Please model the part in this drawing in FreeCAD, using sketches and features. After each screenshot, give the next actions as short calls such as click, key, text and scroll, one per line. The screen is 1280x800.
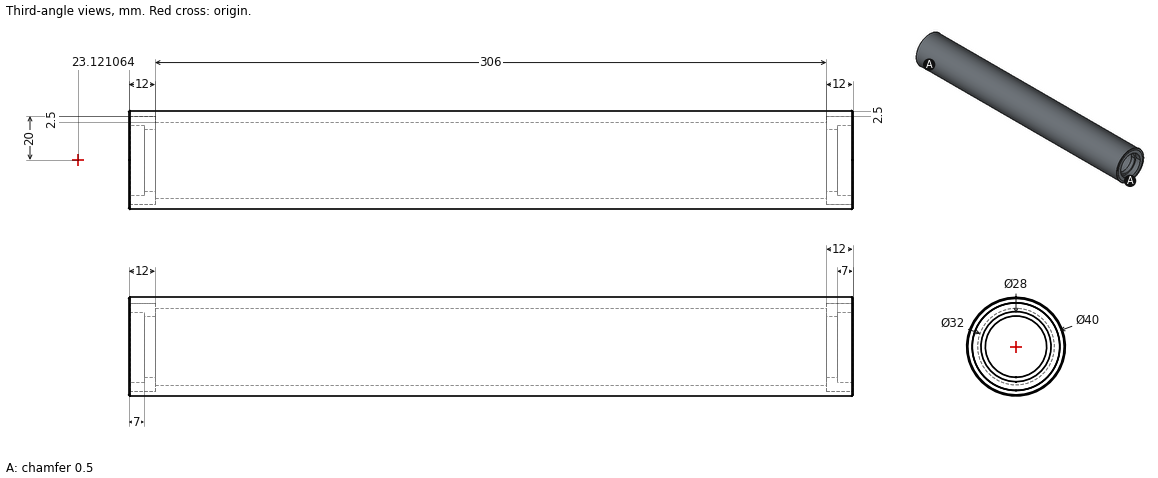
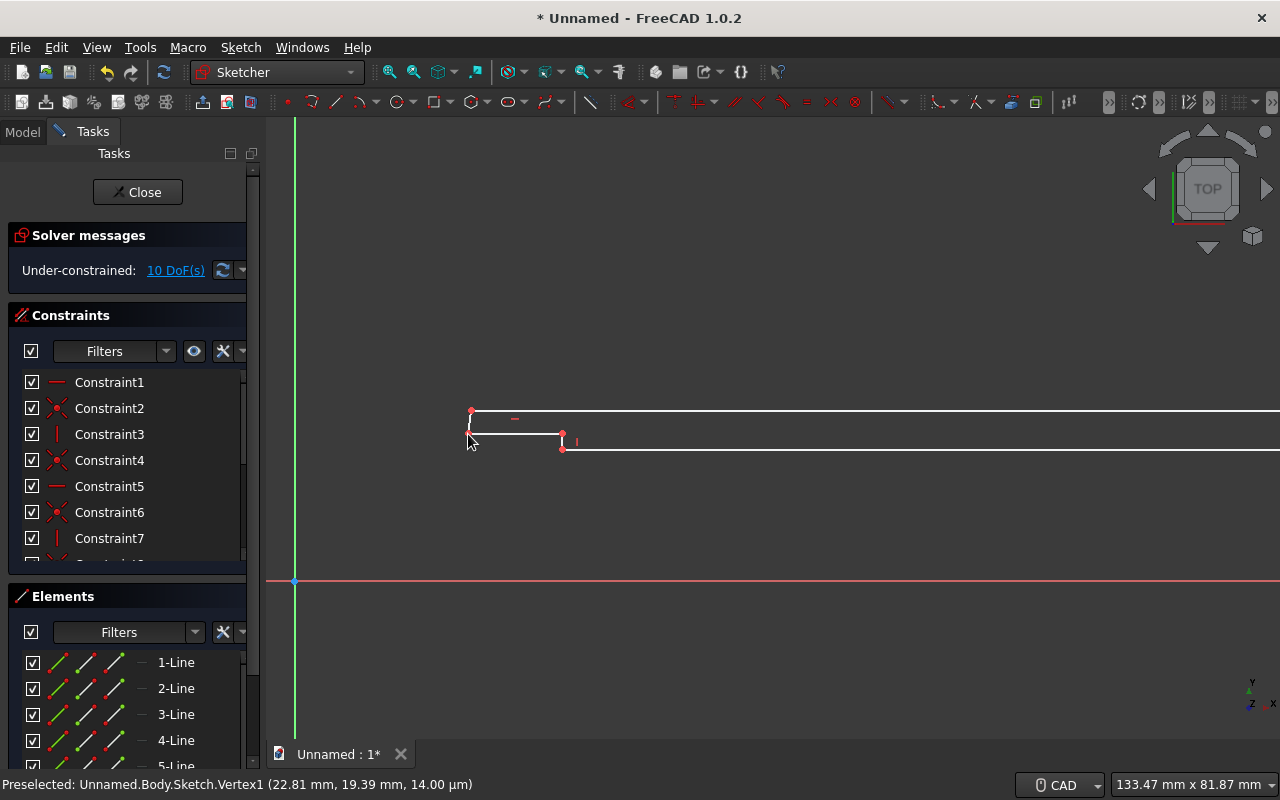
scroll(469, 411, down, 8)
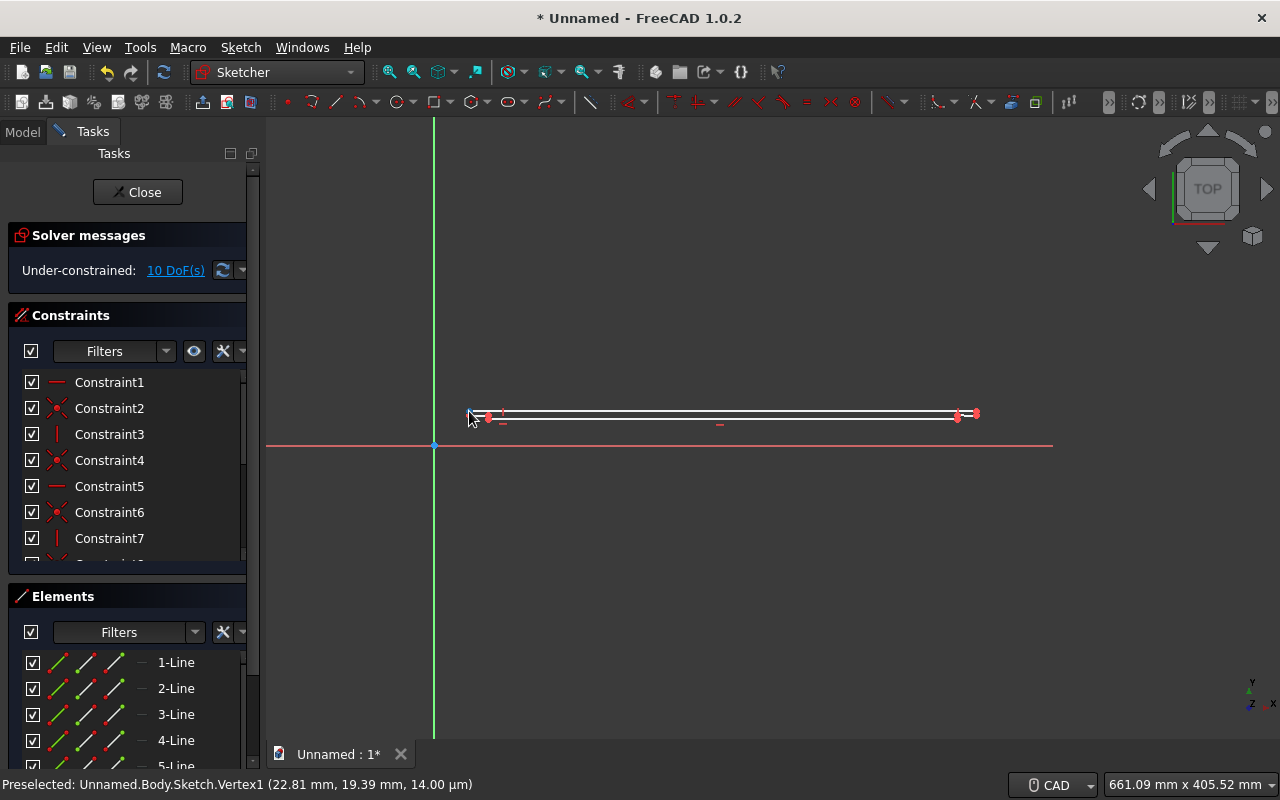
scroll(963, 415, up, 7)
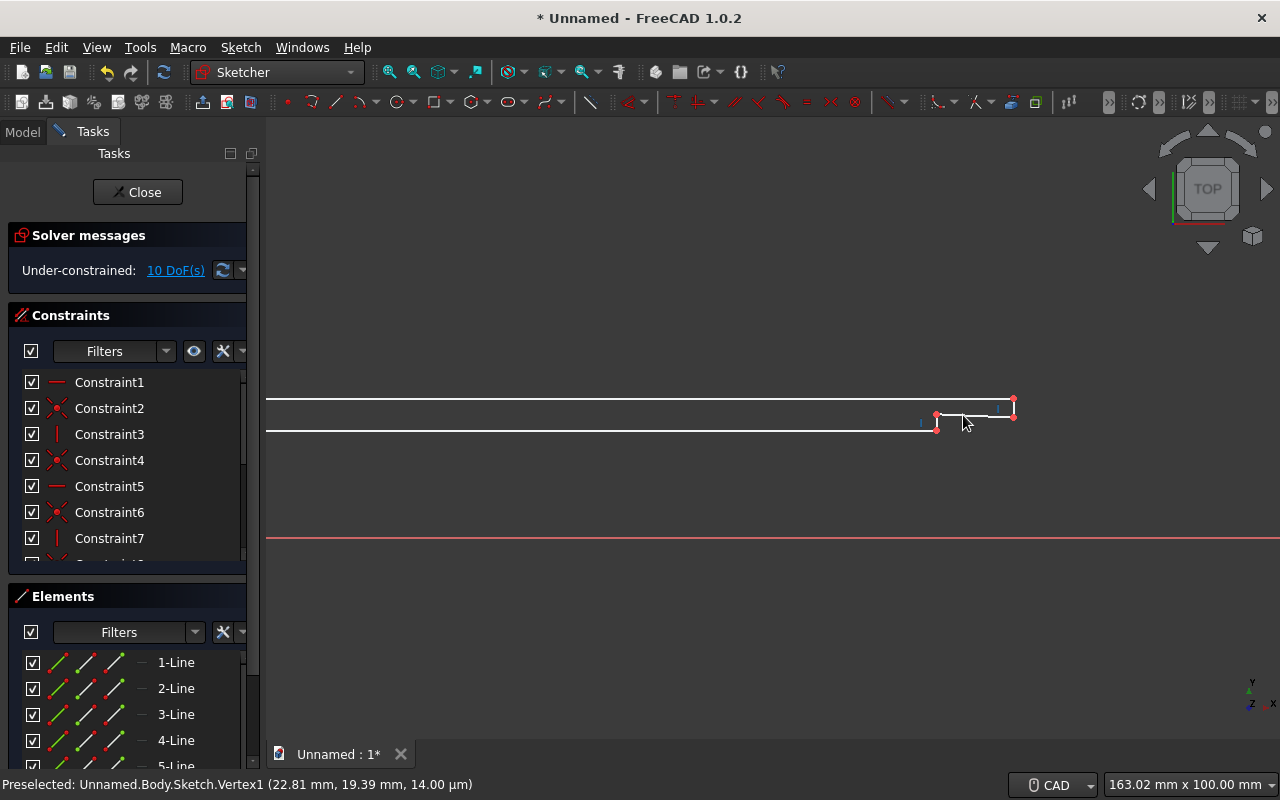
click(960, 415)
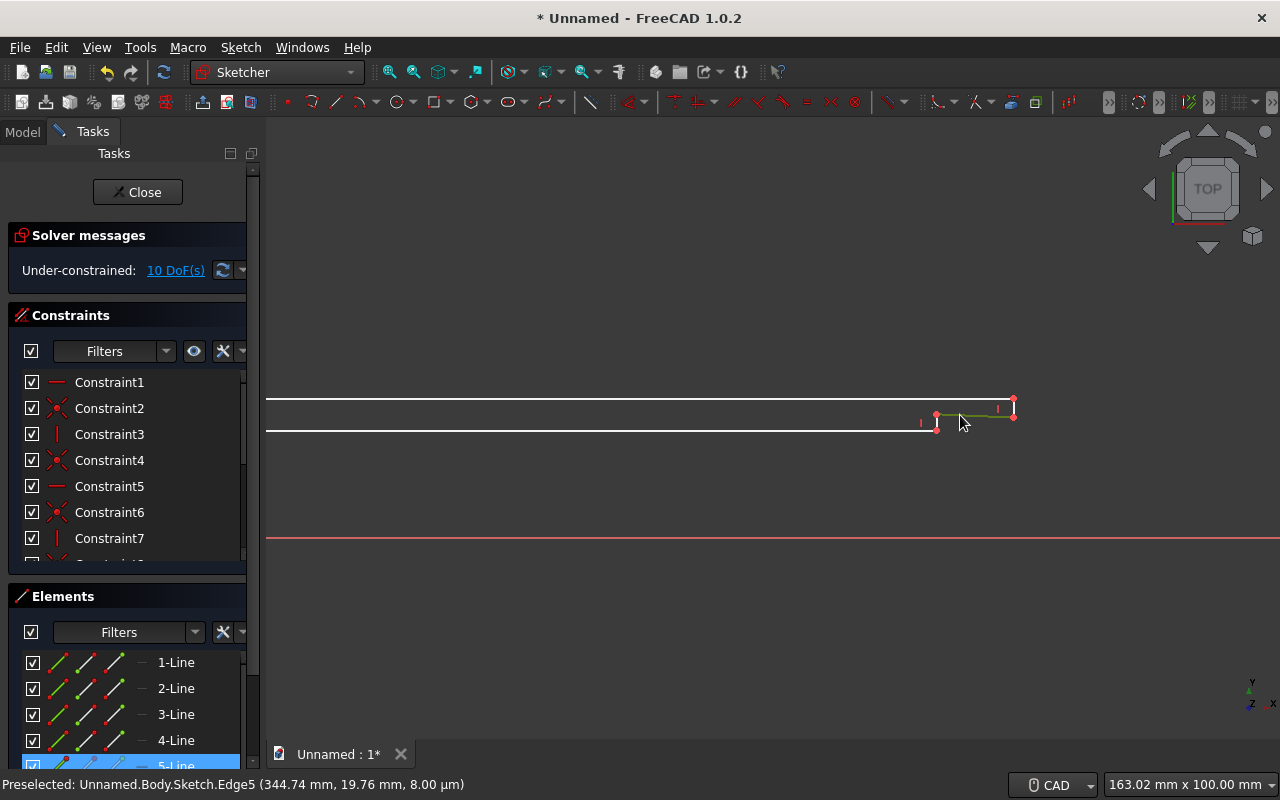
click(716, 102)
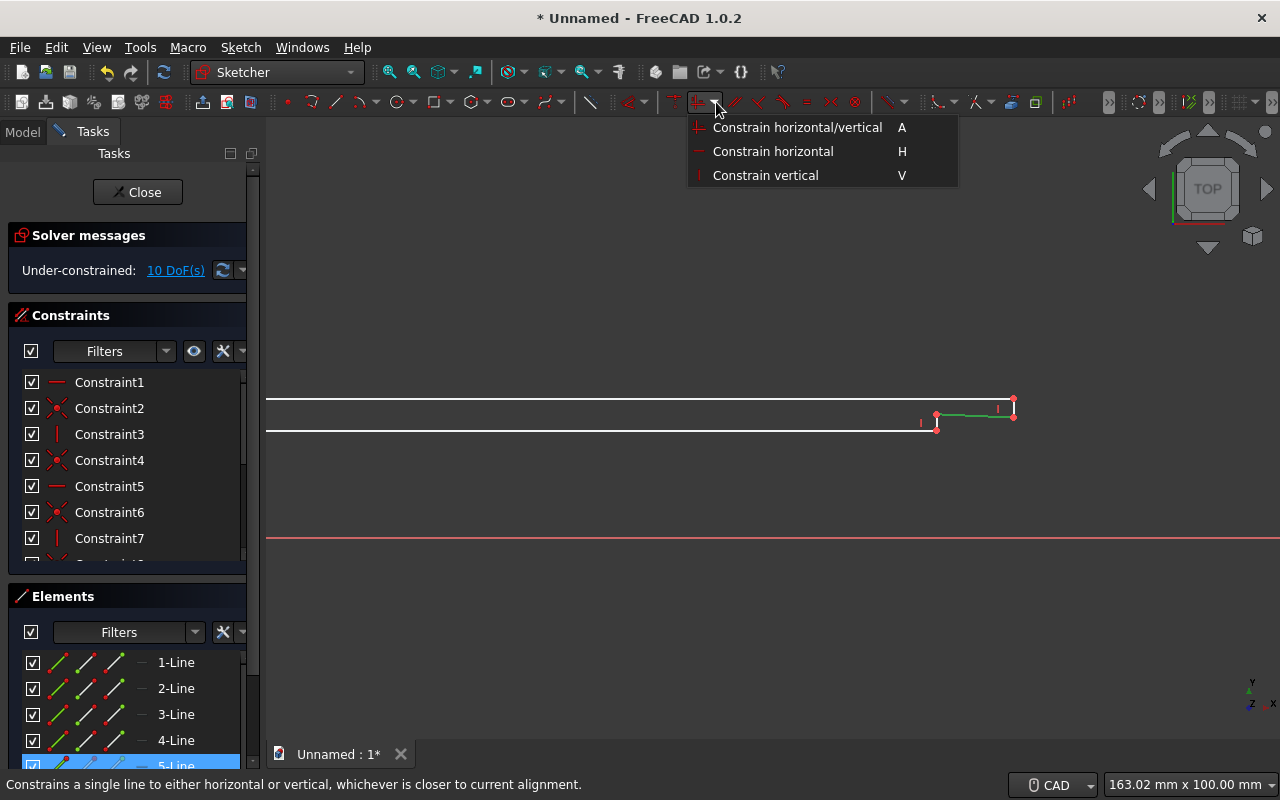
click(823, 151)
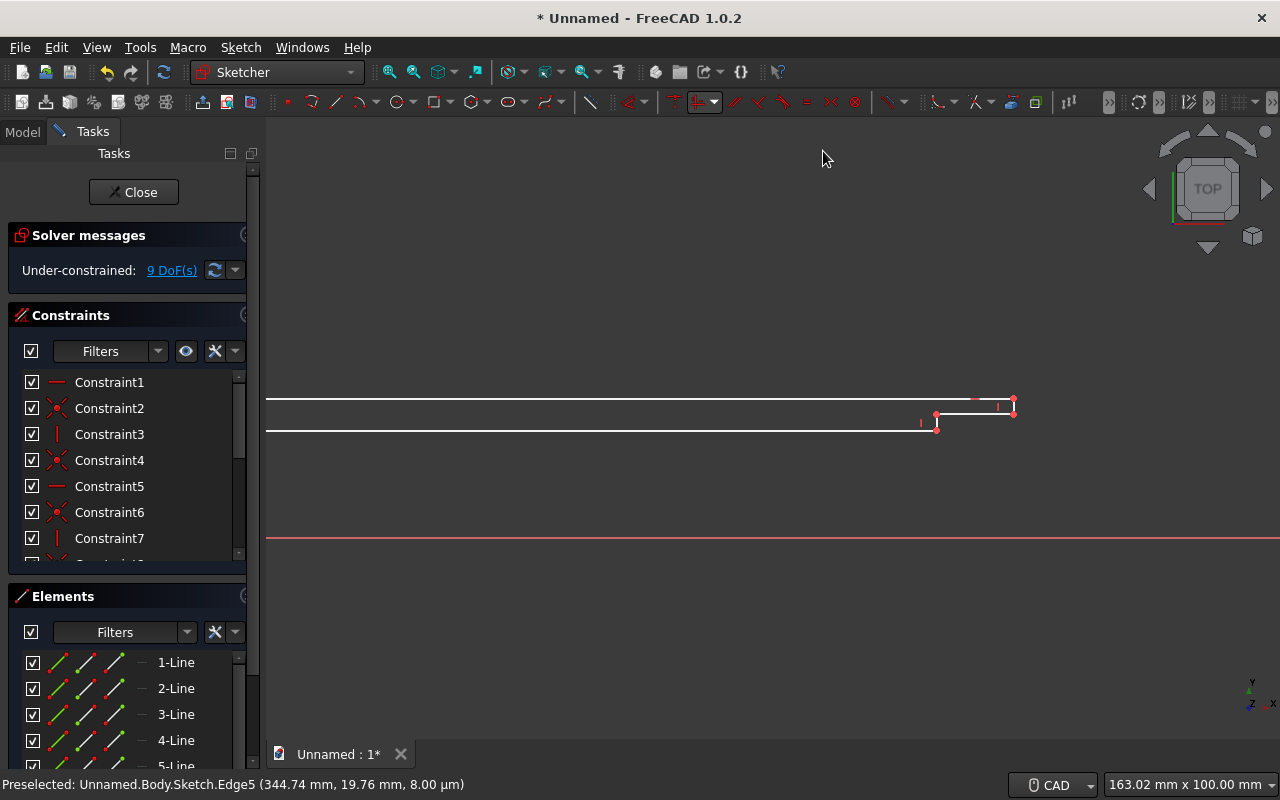
scroll(963, 415, down, 7)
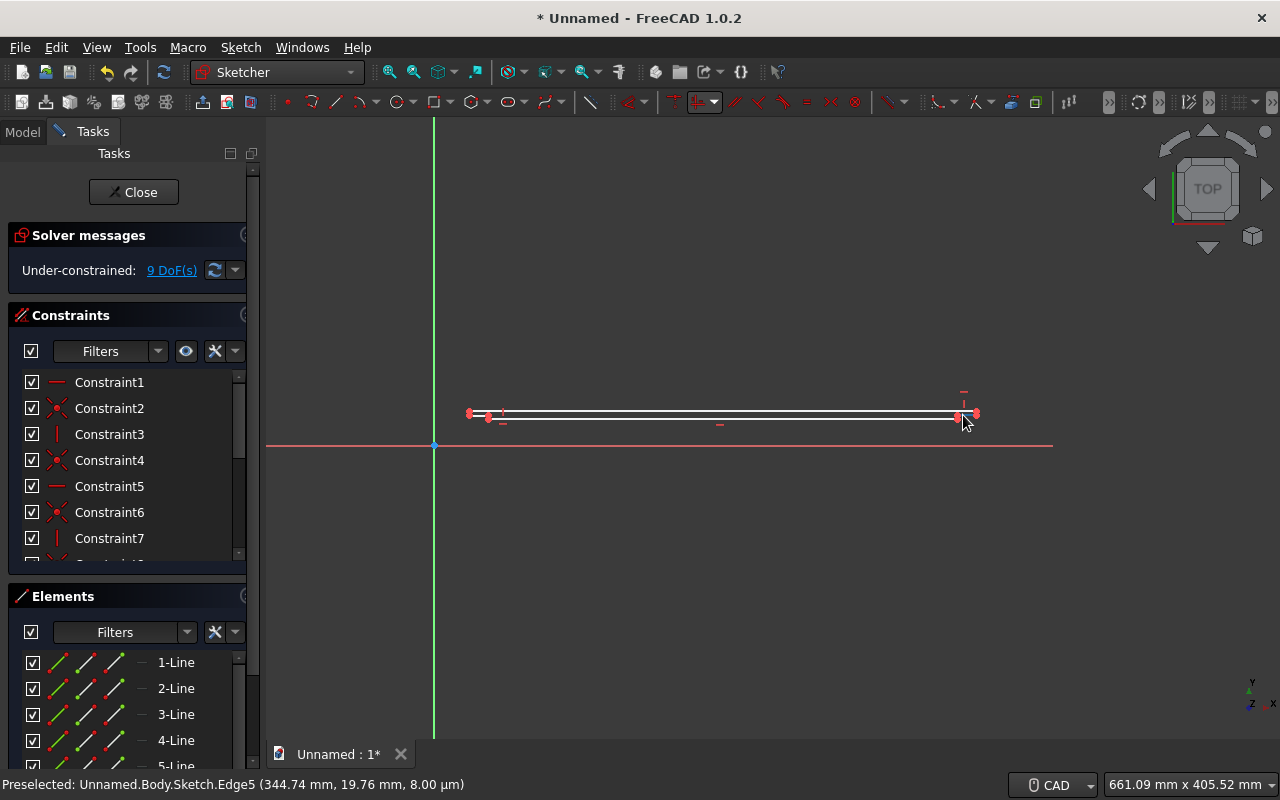
scroll(469, 414, up, 9)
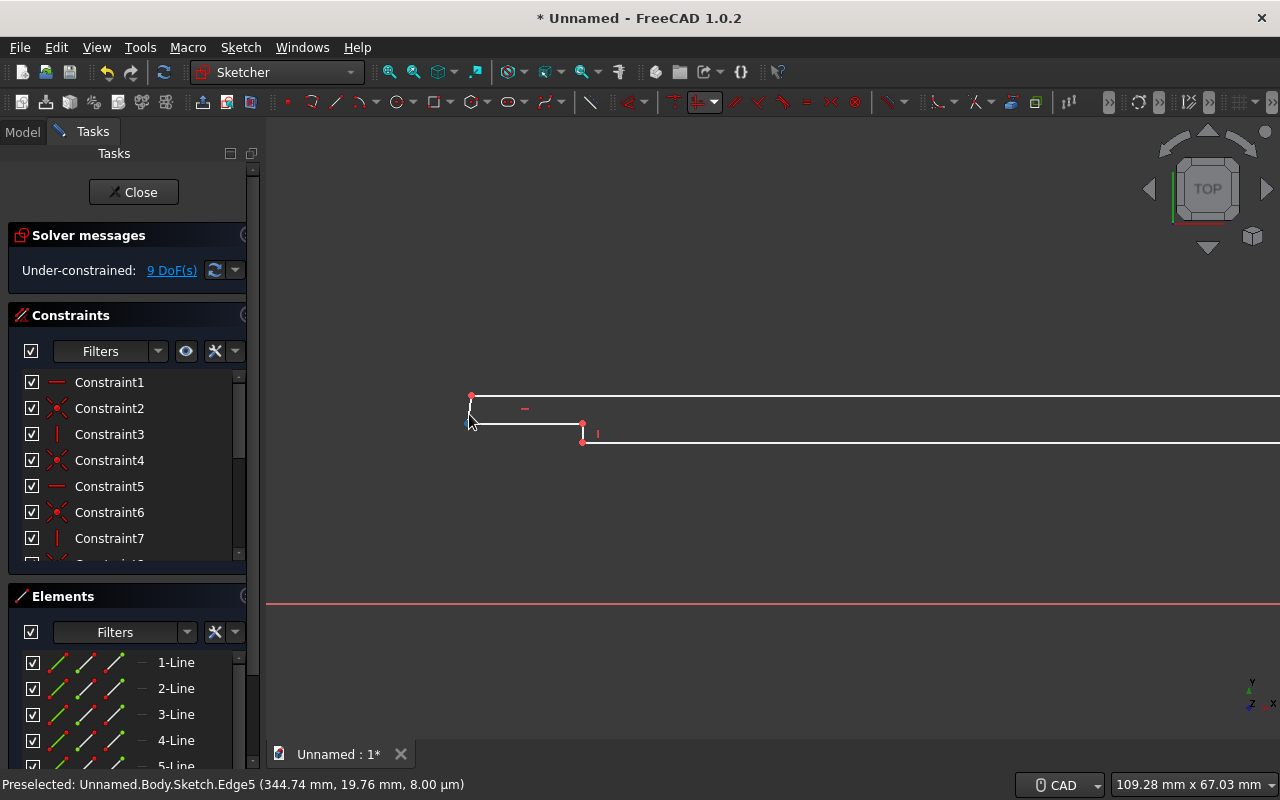
click(470, 410)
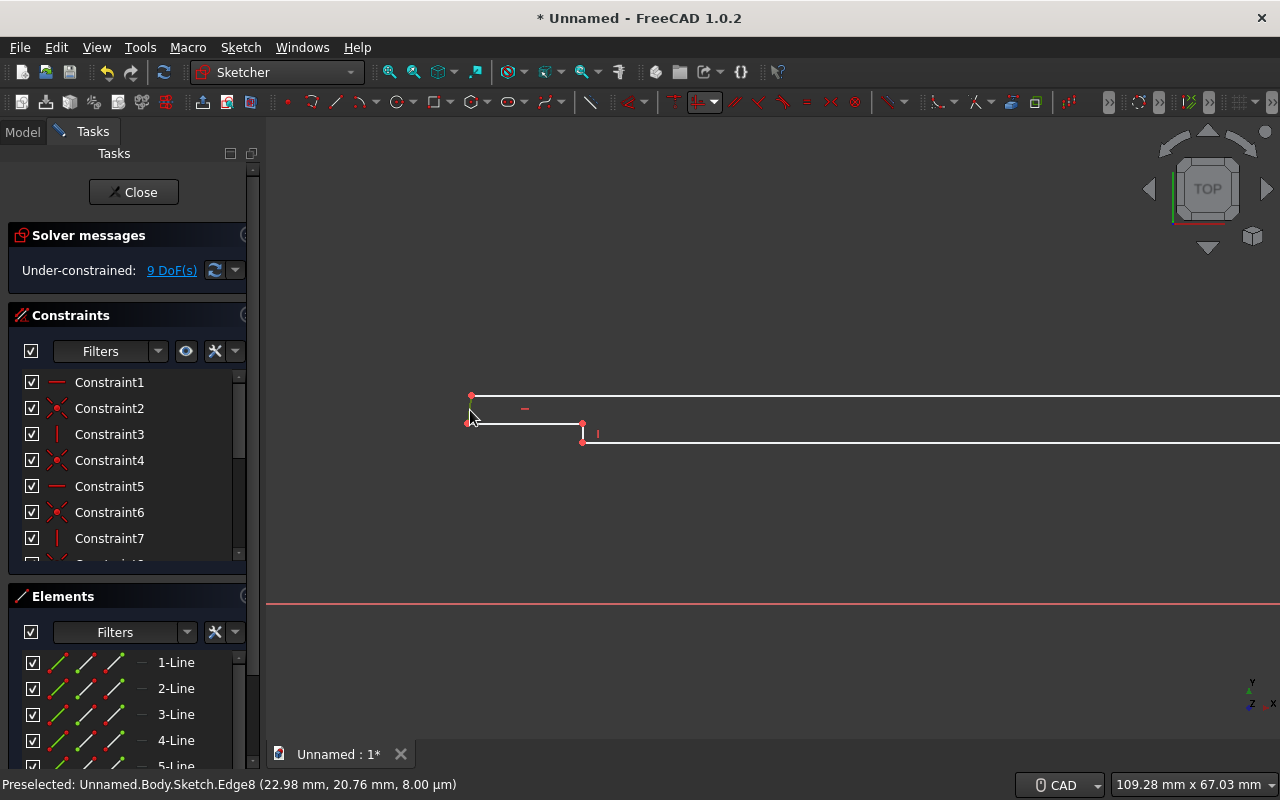
click(716, 102)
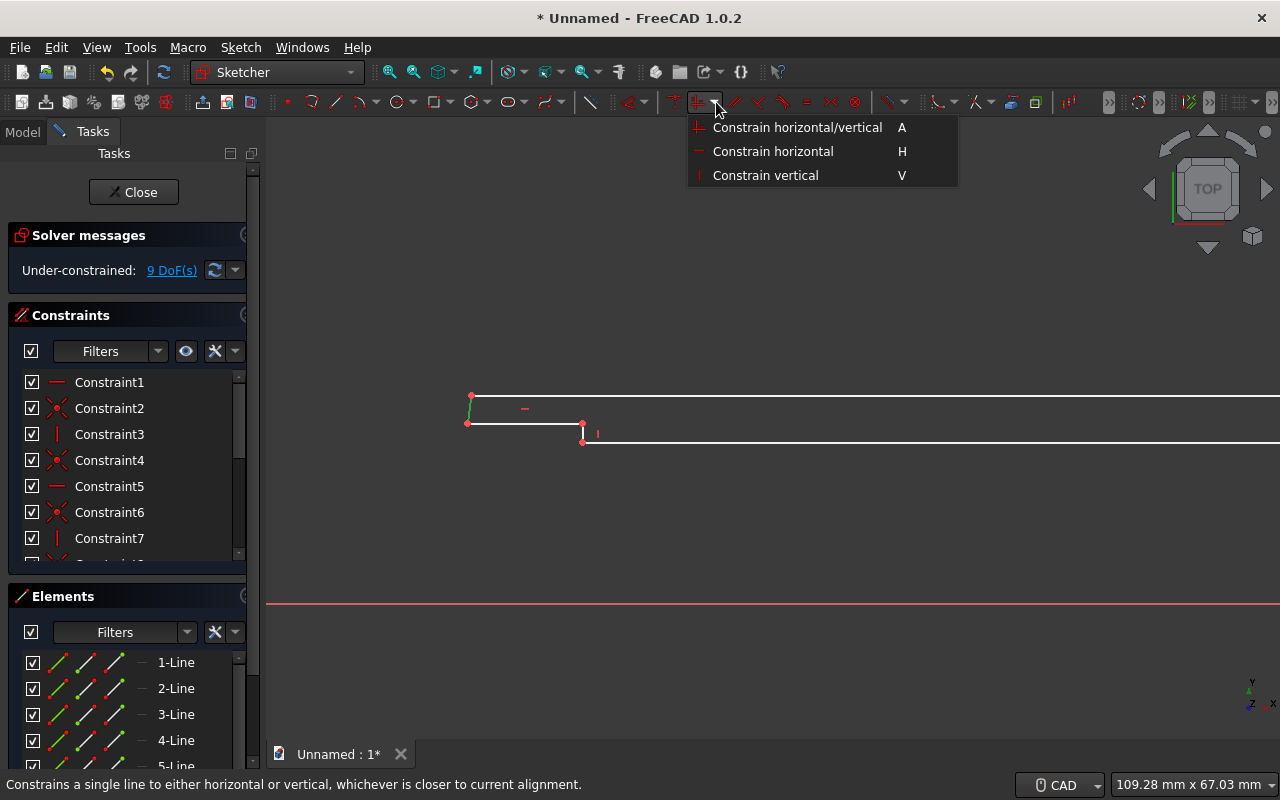
click(823, 175)